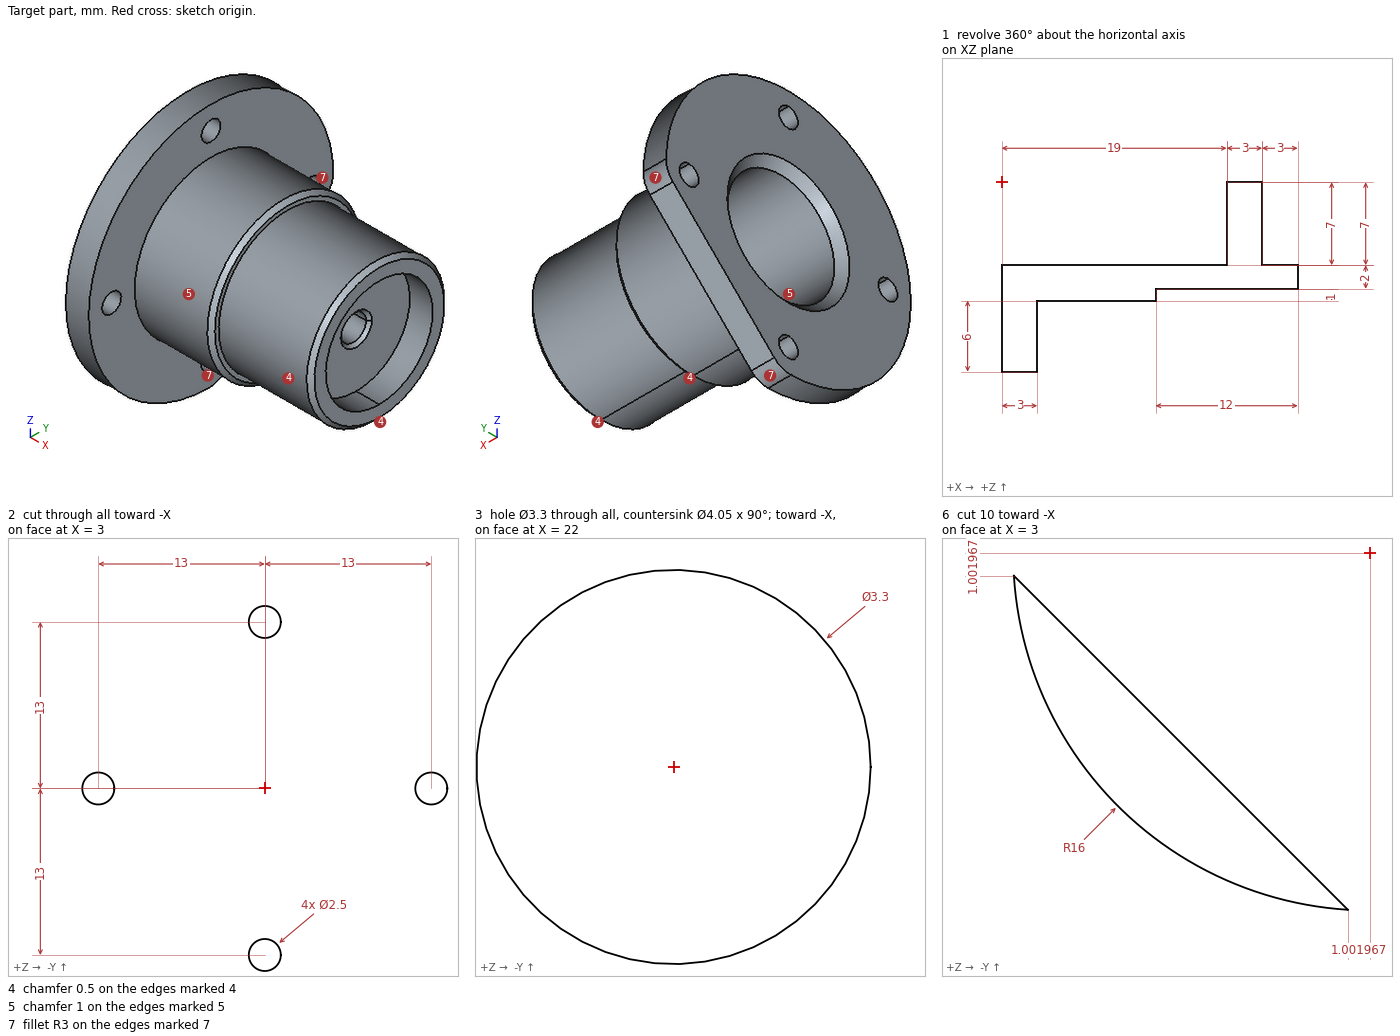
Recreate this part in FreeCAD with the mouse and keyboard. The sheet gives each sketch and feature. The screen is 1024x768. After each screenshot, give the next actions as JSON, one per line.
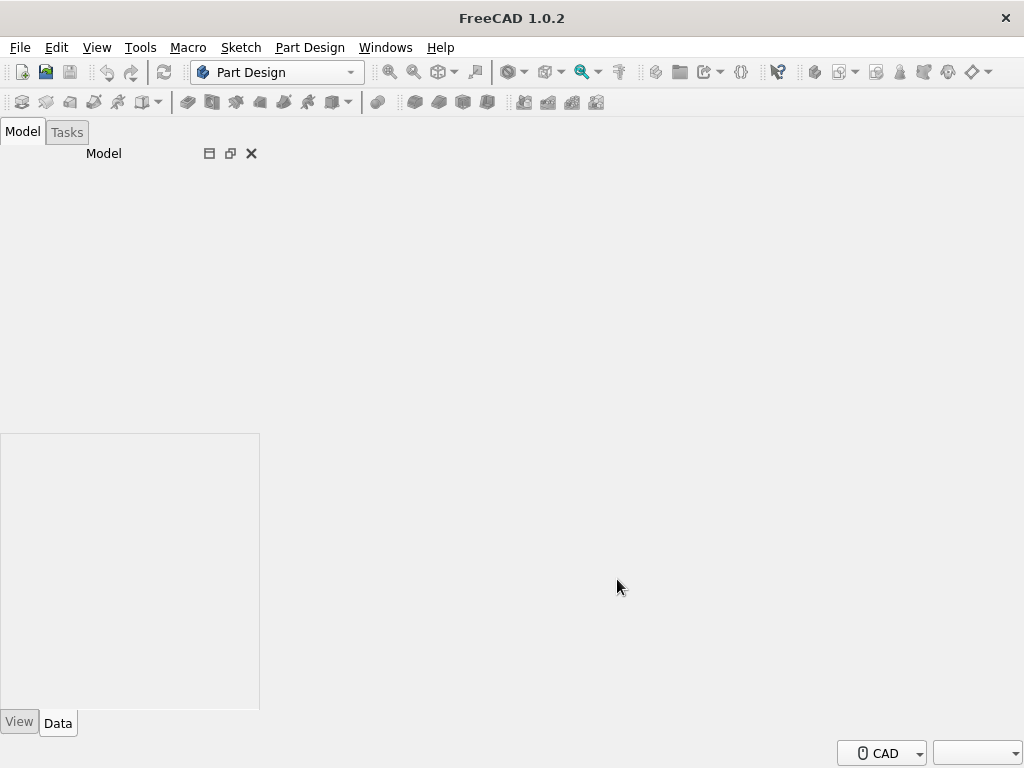
{"action": "left_click", "coordinate": [22, 72]}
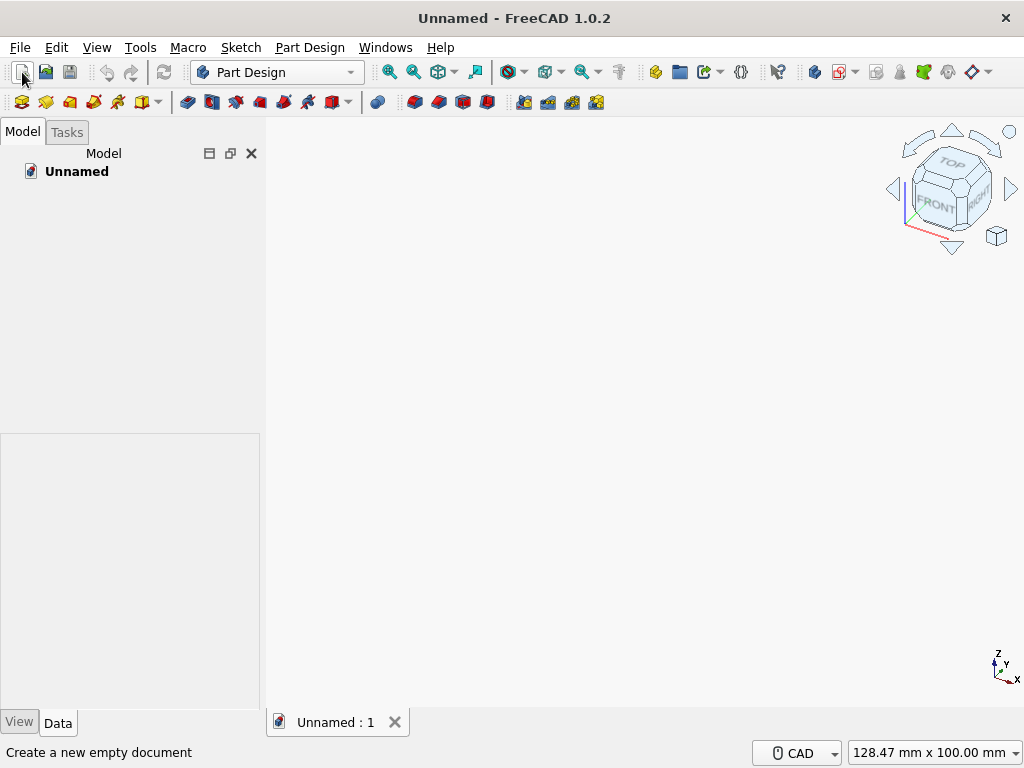
{"action": "left_click", "coordinate": [840, 72]}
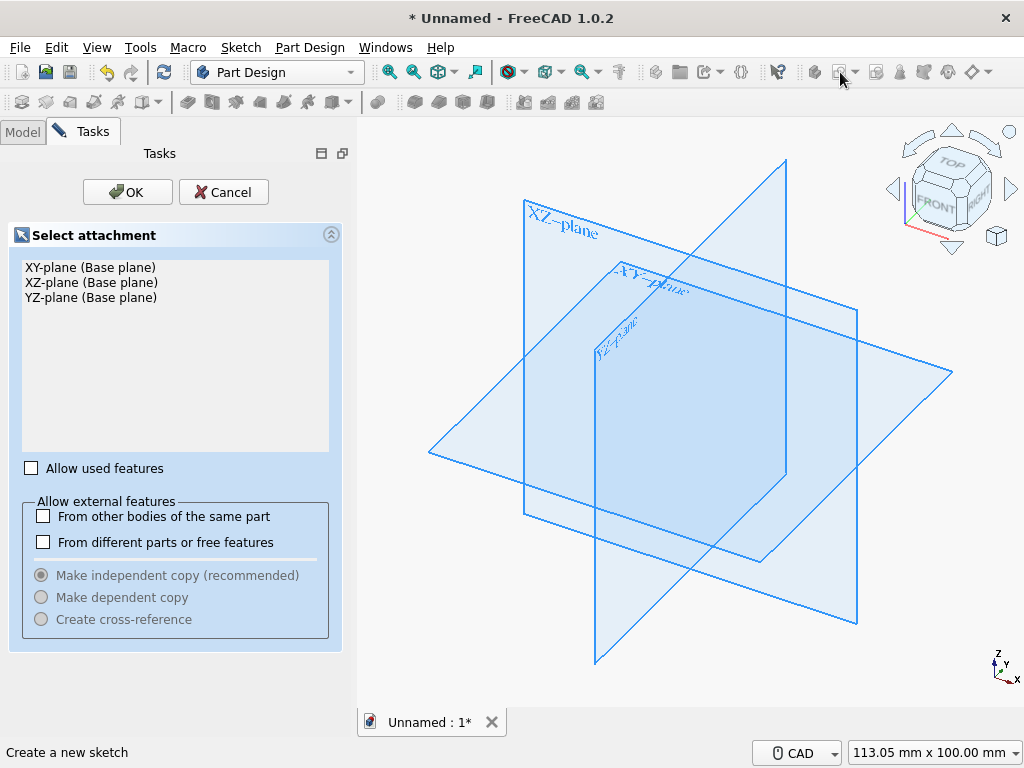
{"action": "left_click", "coordinate": [82, 282]}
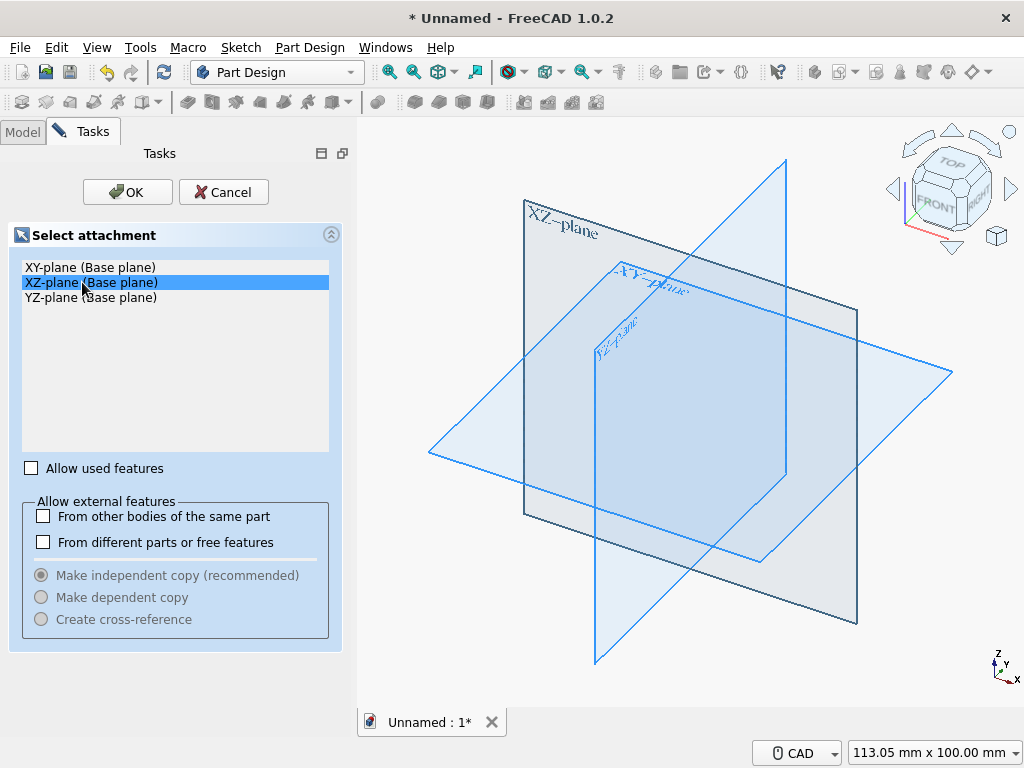
{"action": "left_click", "coordinate": [128, 192]}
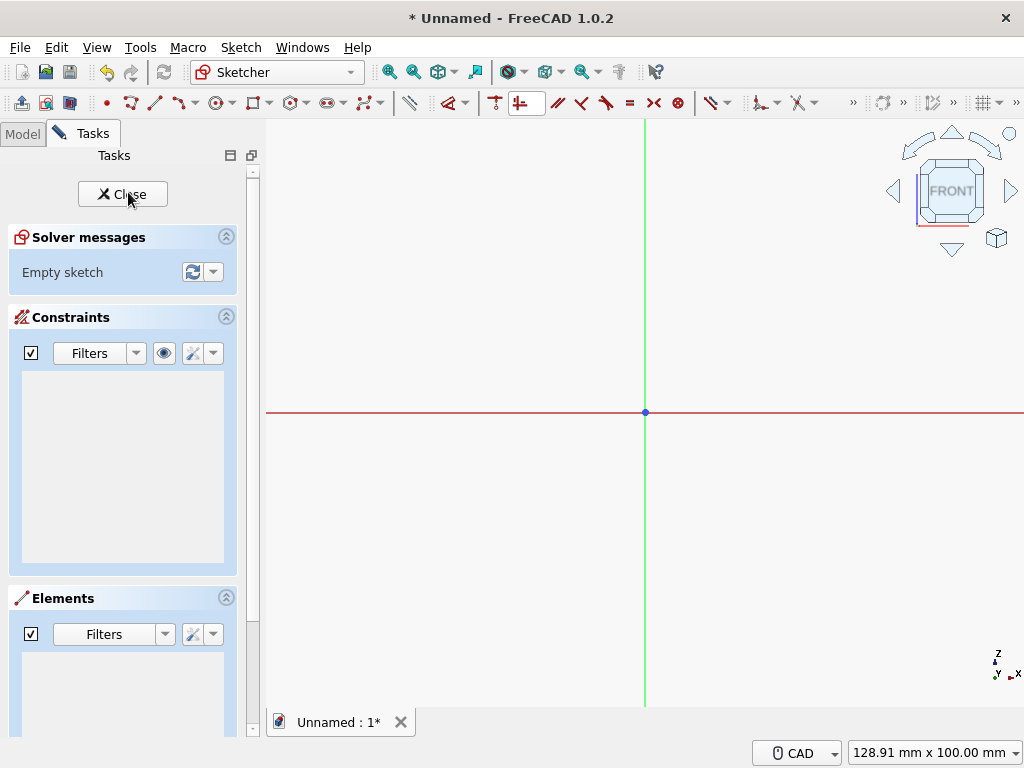
{"action": "scroll", "coordinate": [801, 487], "scroll_direction": "up", "scroll_amount": 5}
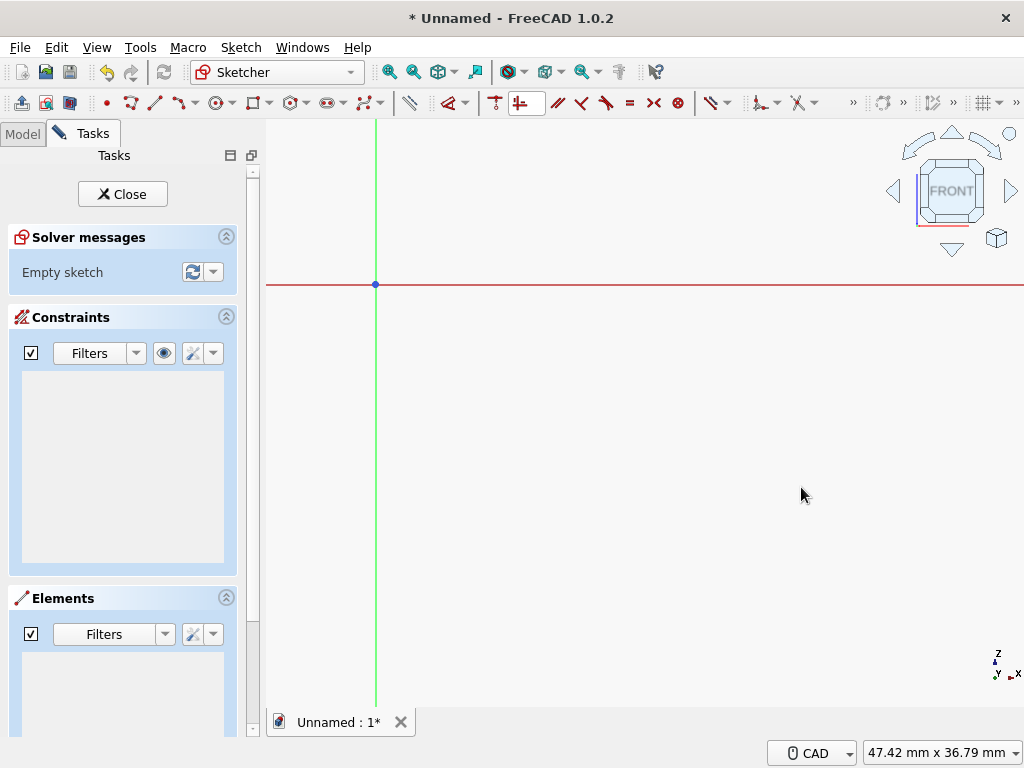
{"action": "key", "text": "g m"}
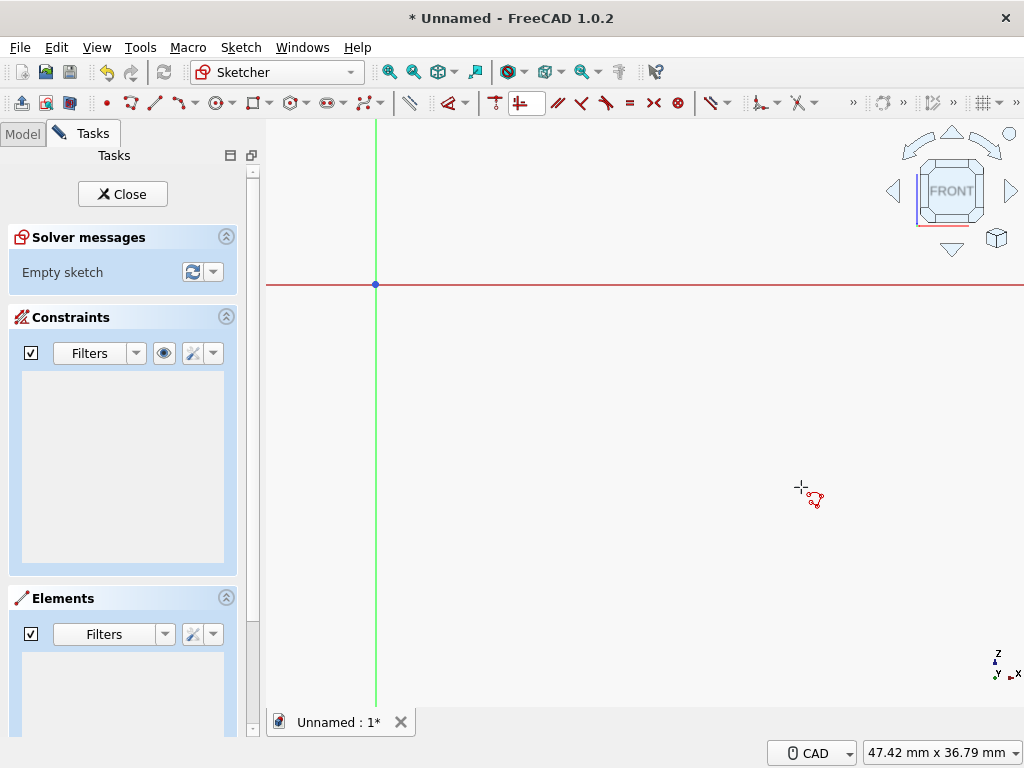
{"action": "left_click", "coordinate": [376, 397]}
{"action": "left_click", "coordinate": [679, 397]}
{"action": "left_click", "coordinate": [679, 285]}
{"action": "left_click", "coordinate": [727, 294]}
{"action": "left_click", "coordinate": [727, 397]}
{"action": "left_click", "coordinate": [775, 397]}
{"action": "left_click", "coordinate": [775, 429]}
{"action": "left_click", "coordinate": [584, 429]}
{"action": "left_click", "coordinate": [584, 445]}
{"action": "left_click", "coordinate": [424, 445]}
{"action": "left_click", "coordinate": [424, 541]}
{"action": "left_click", "coordinate": [385, 541]}
{"action": "left_click", "coordinate": [376, 398]}
{"action": "key", "text": "Escape"}
{"action": "key", "text": "Escape"}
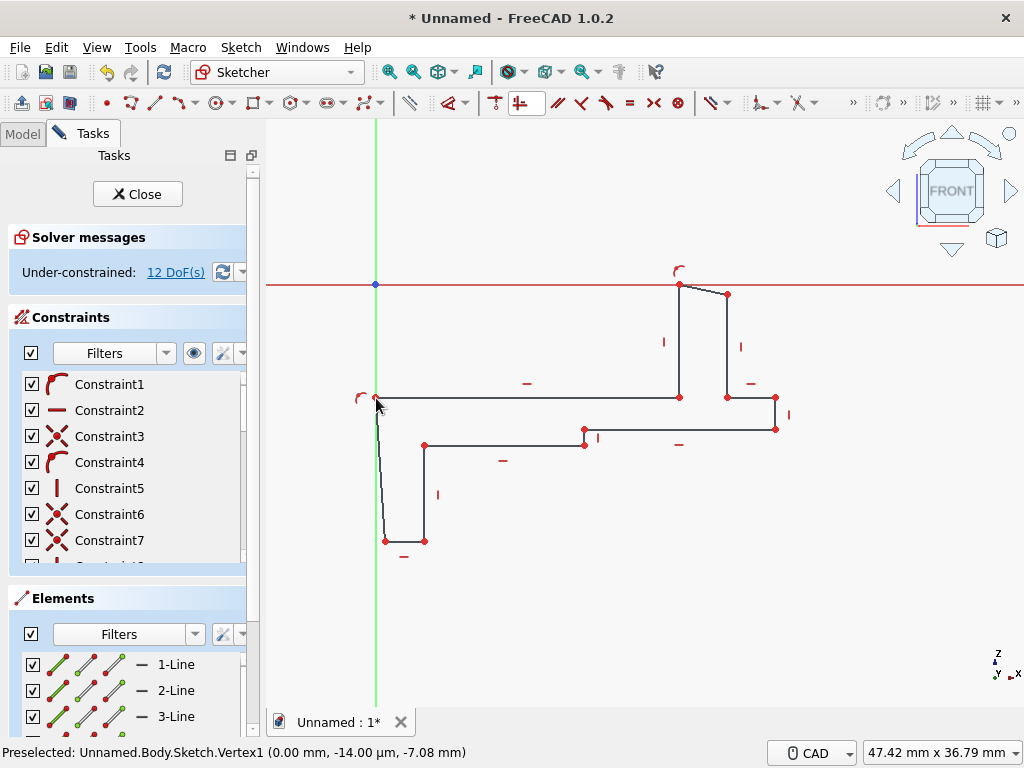
{"action": "left_click", "coordinate": [693, 288]}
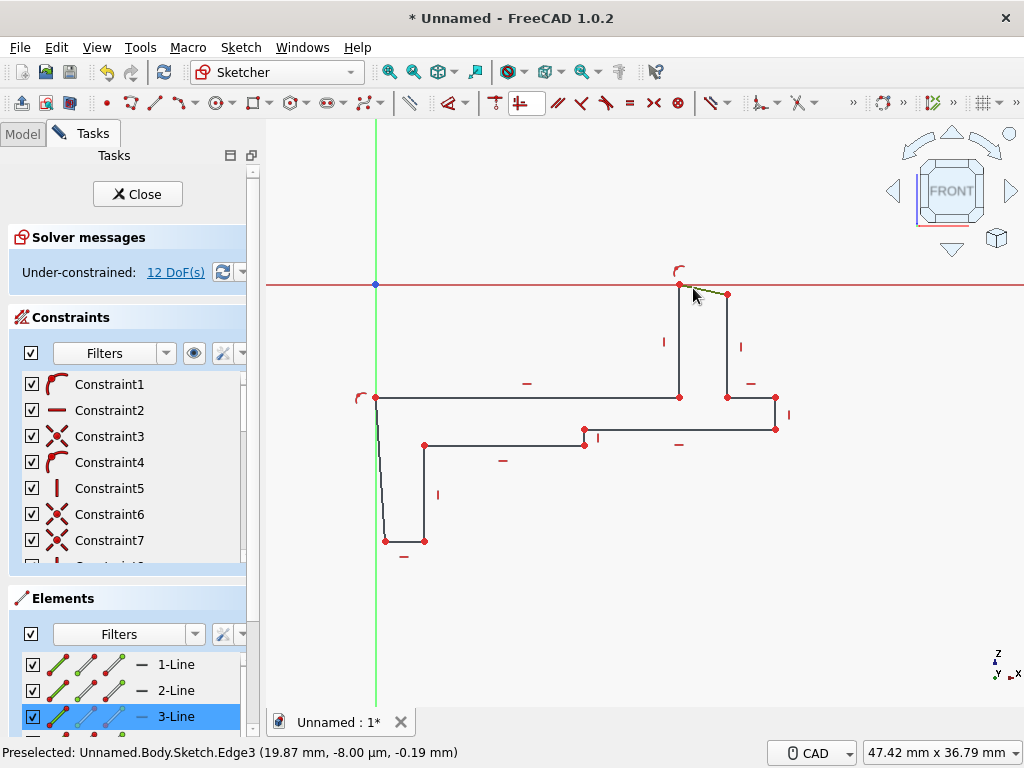
{"action": "key", "text": "h"}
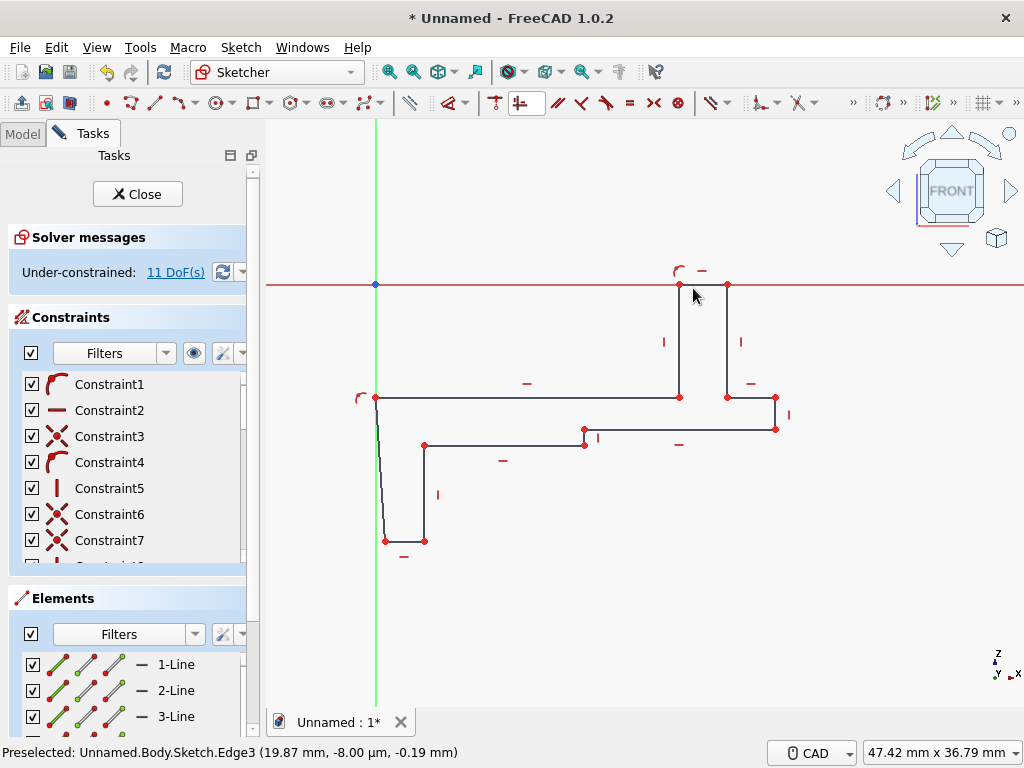
{"action": "left_click", "coordinate": [379, 441]}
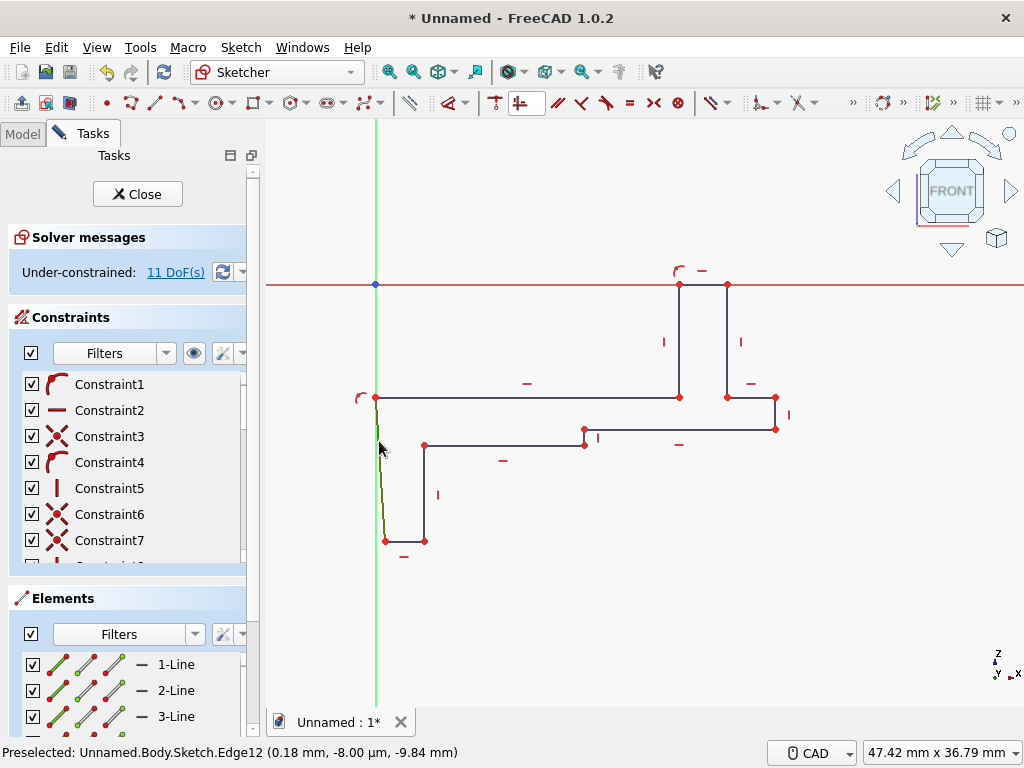
{"action": "left_click", "coordinate": [540, 104]}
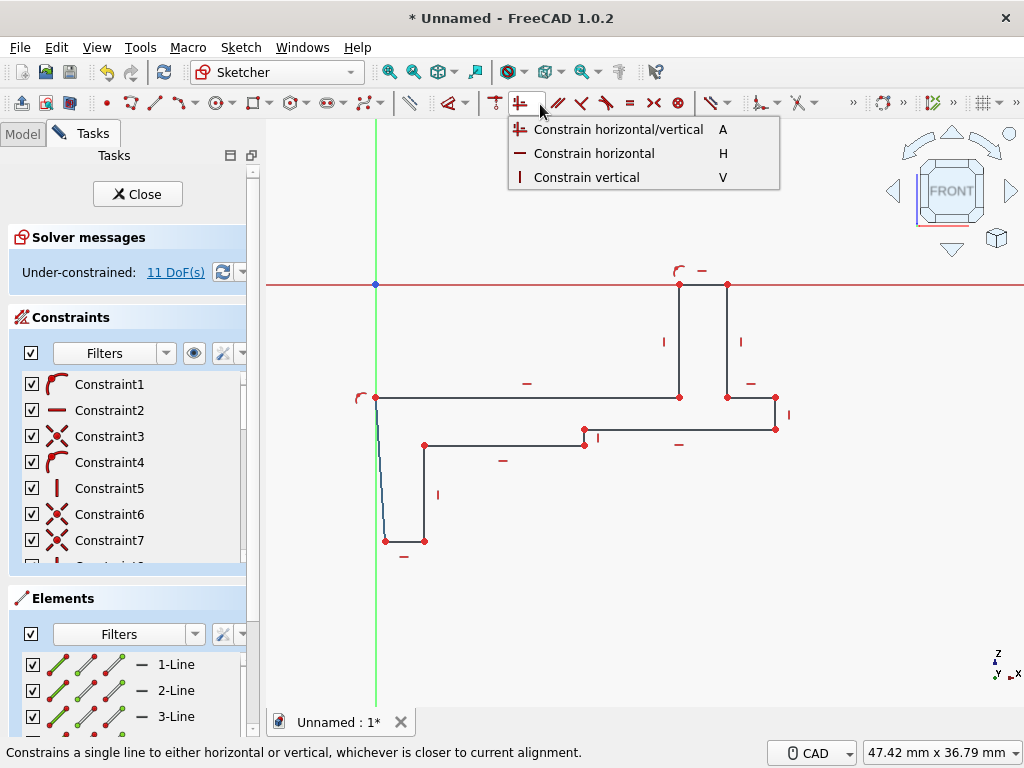
{"action": "left_click", "coordinate": [644, 177]}